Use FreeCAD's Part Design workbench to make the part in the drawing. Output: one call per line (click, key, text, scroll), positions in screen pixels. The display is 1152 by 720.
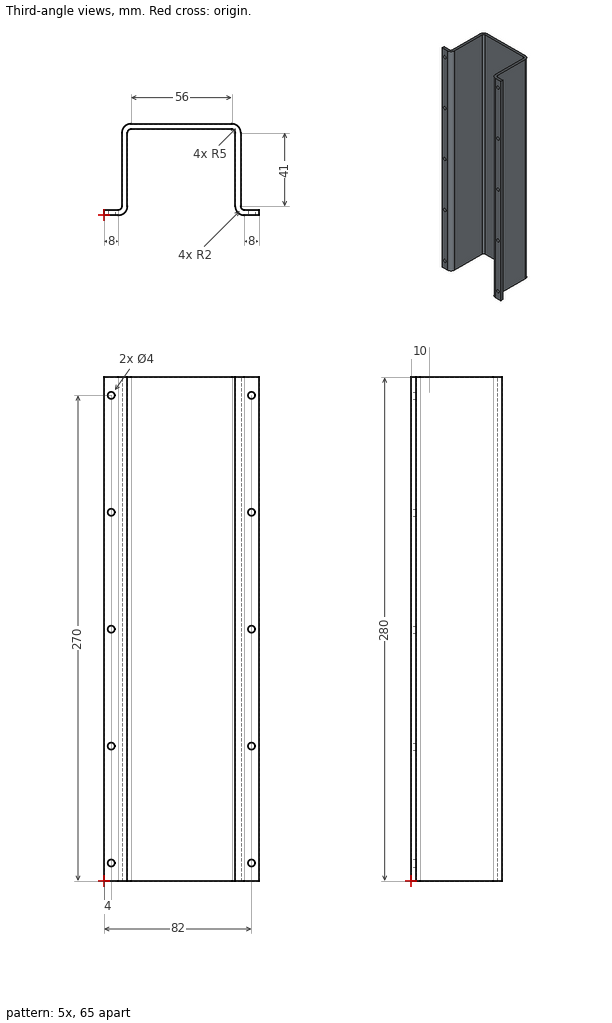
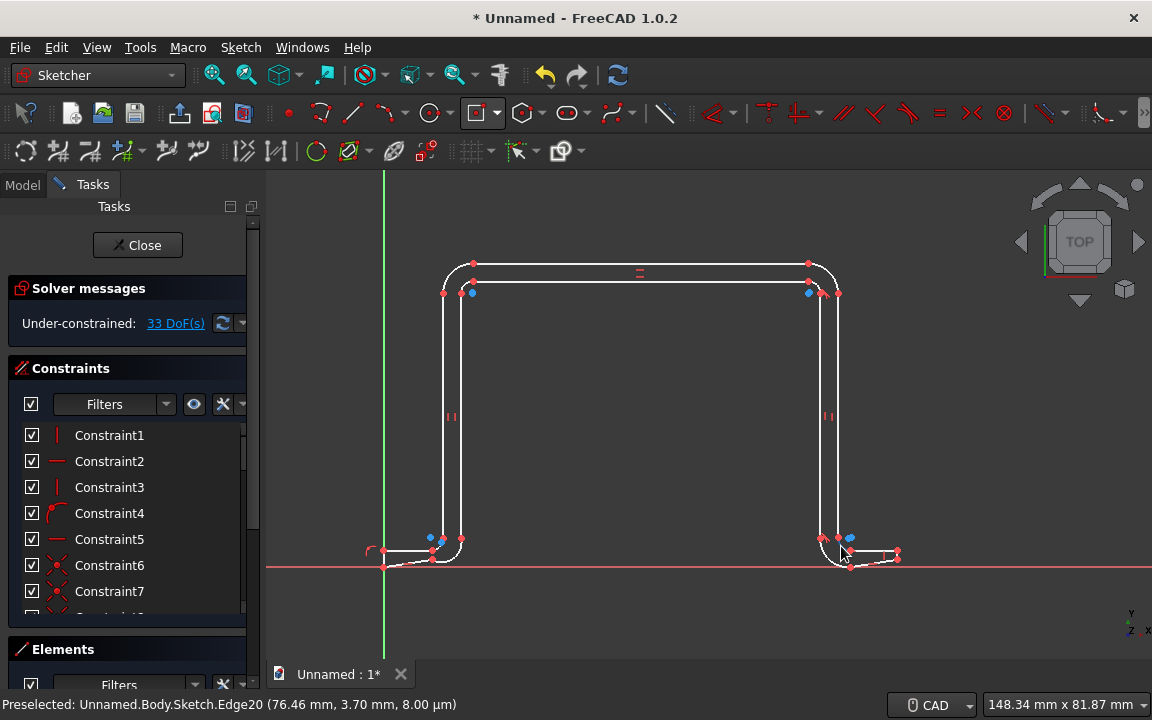
click(708, 264)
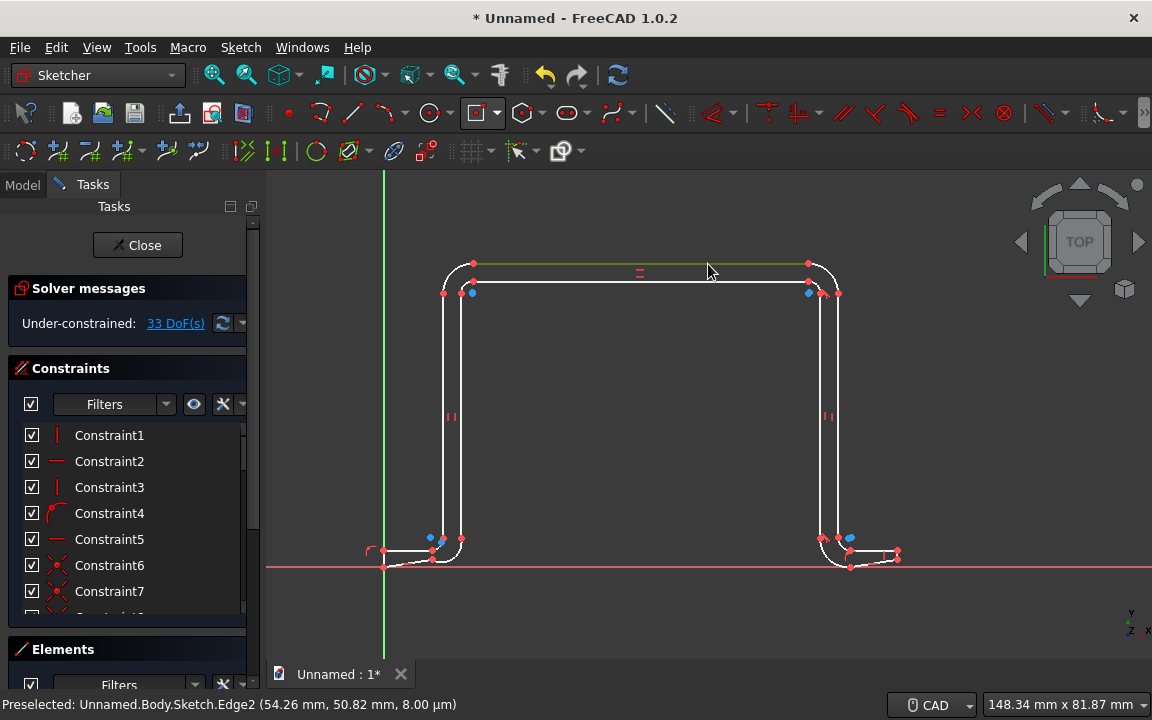
click(835, 280)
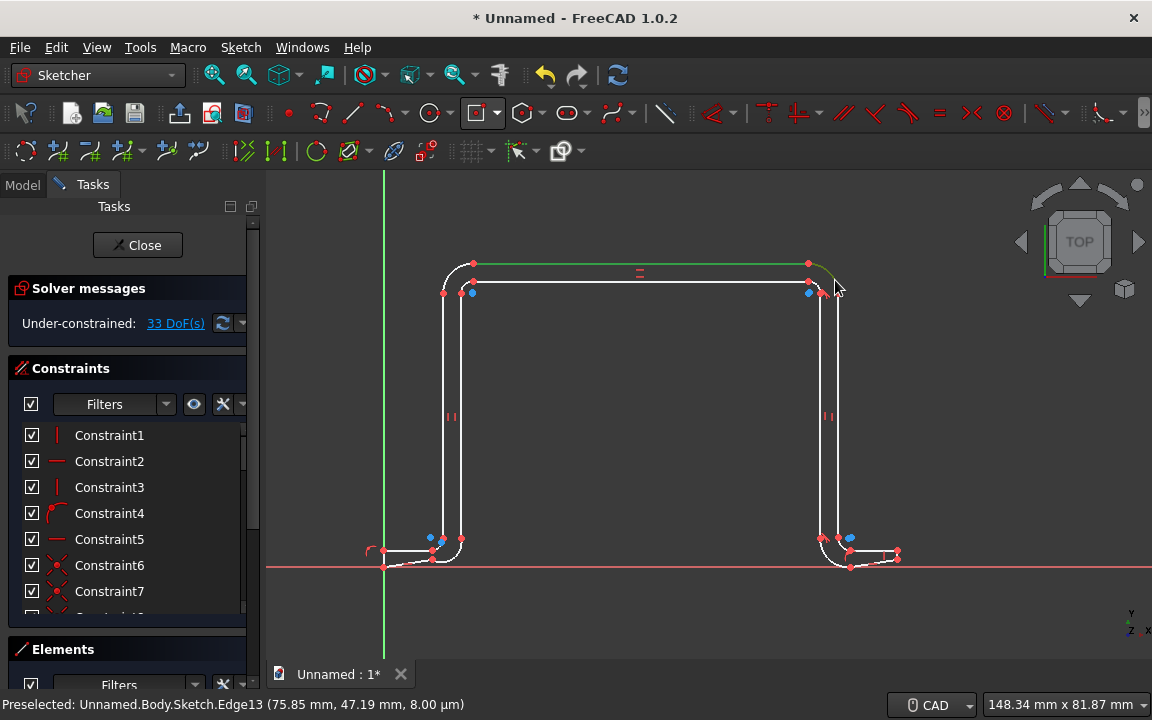
click(908, 114)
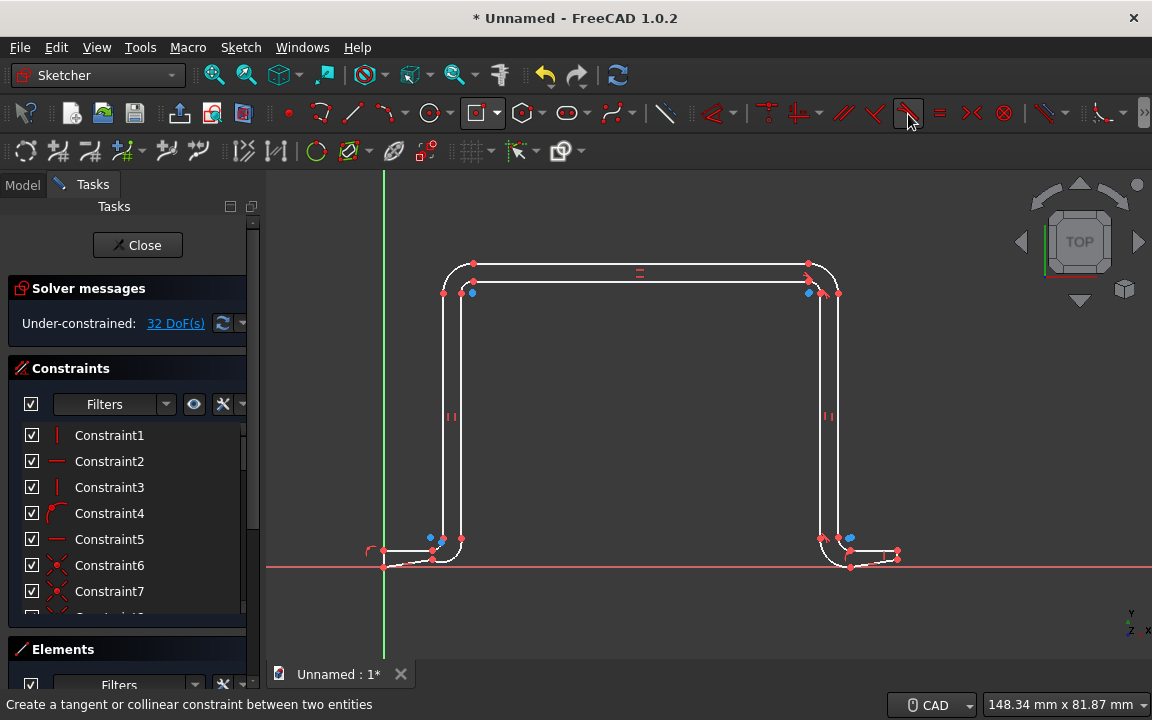
click(708, 264)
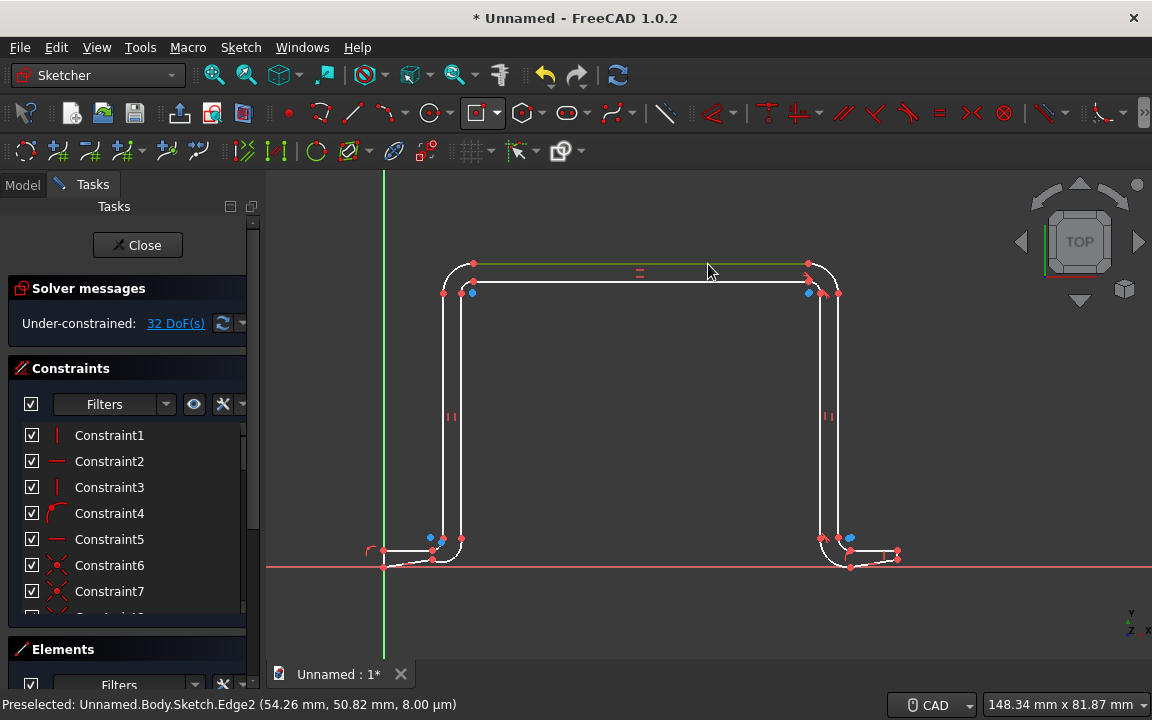
click(459, 267)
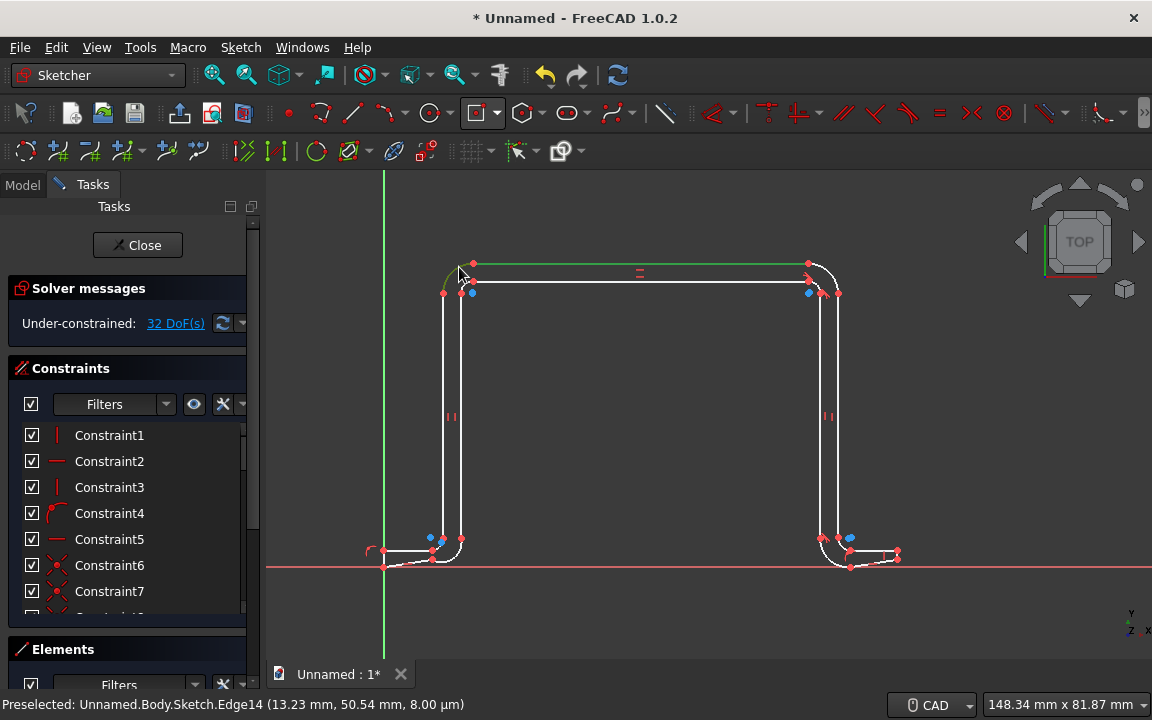
click(908, 114)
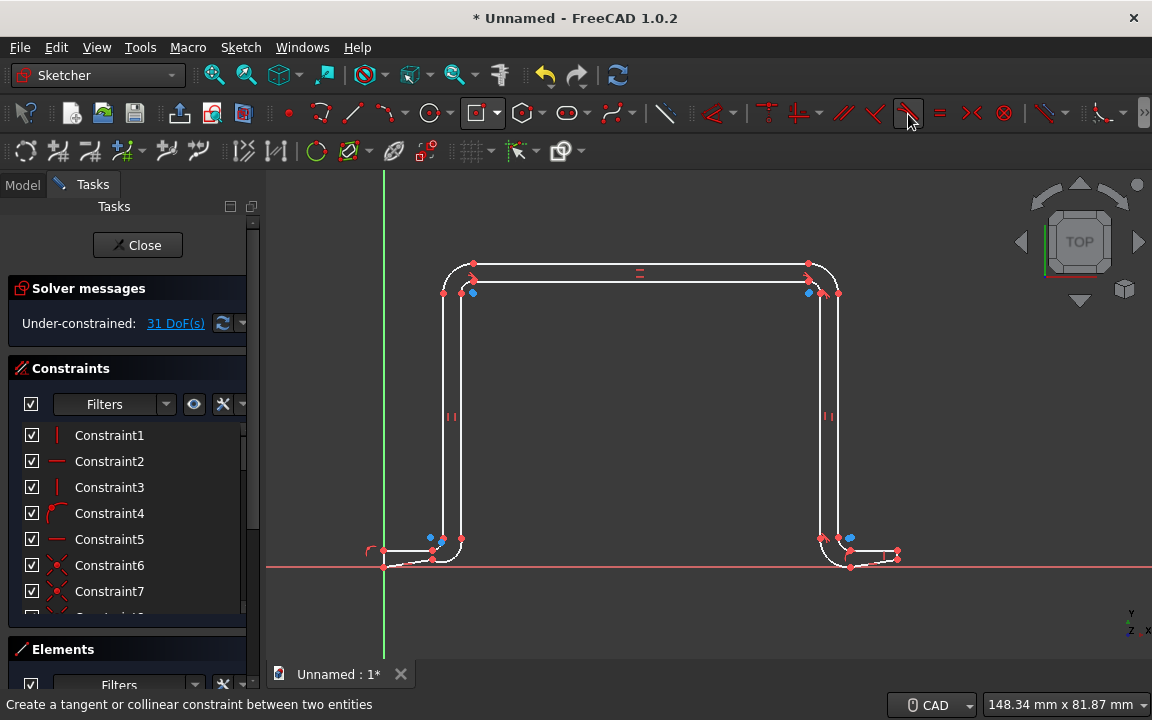
click(443, 367)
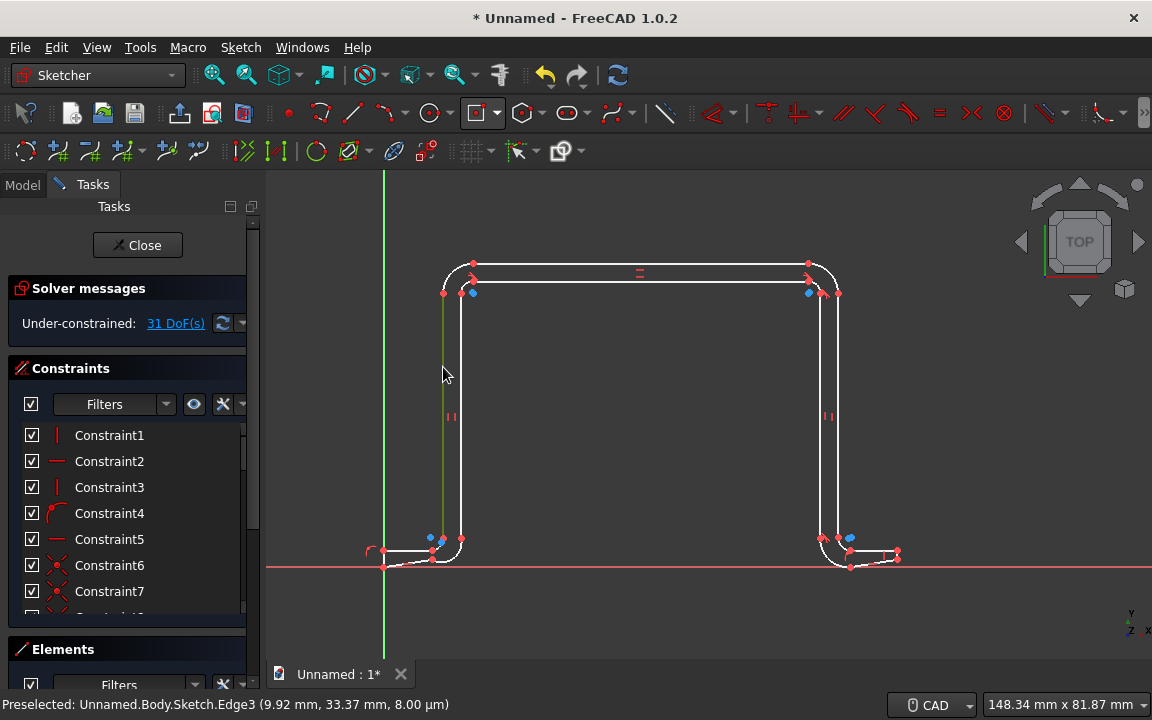
click(460, 267)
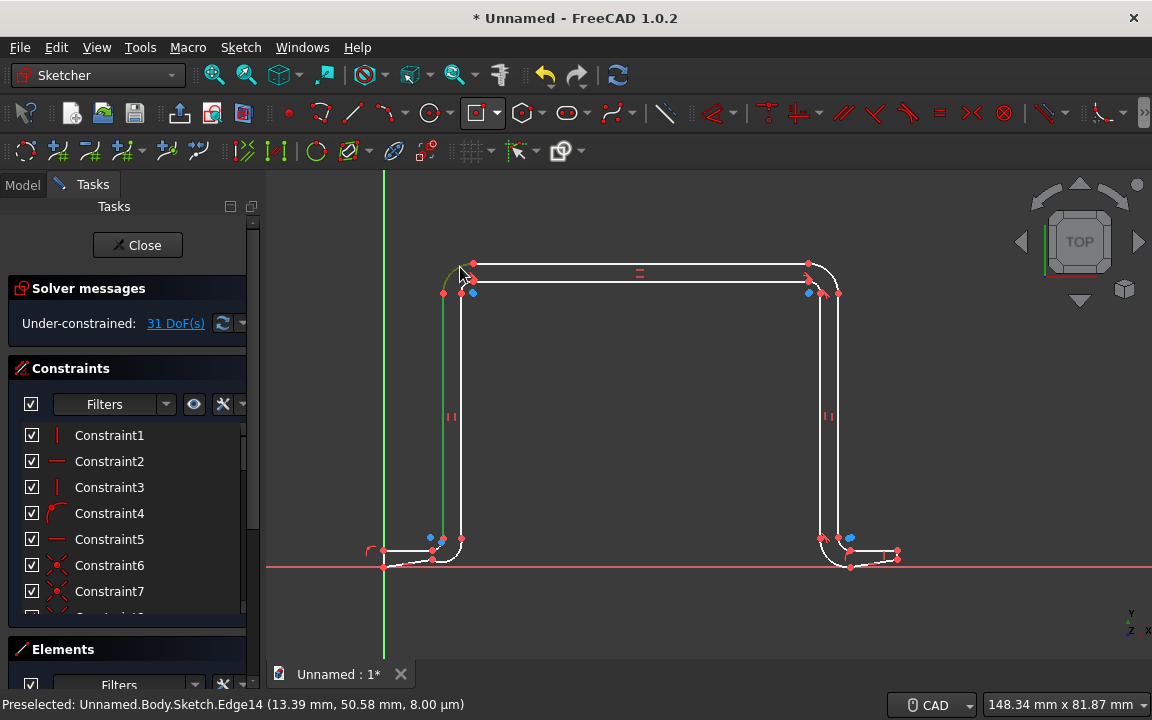
key(t)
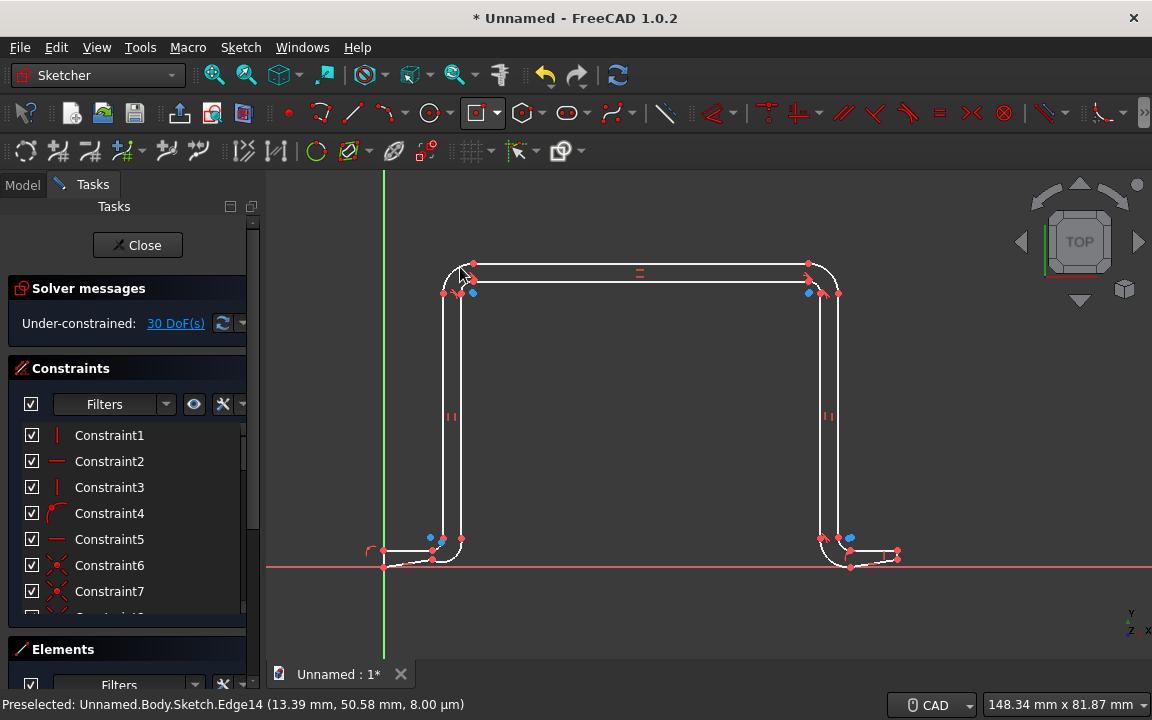
click(443, 367)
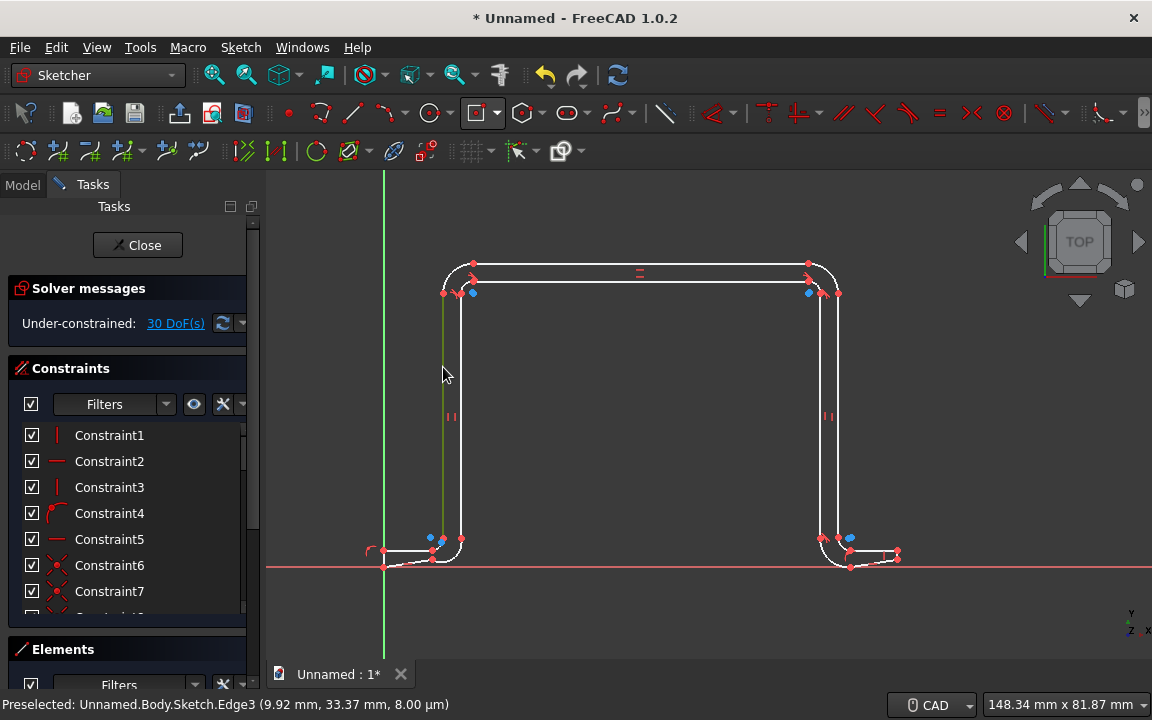
scroll(440, 547, up, 3)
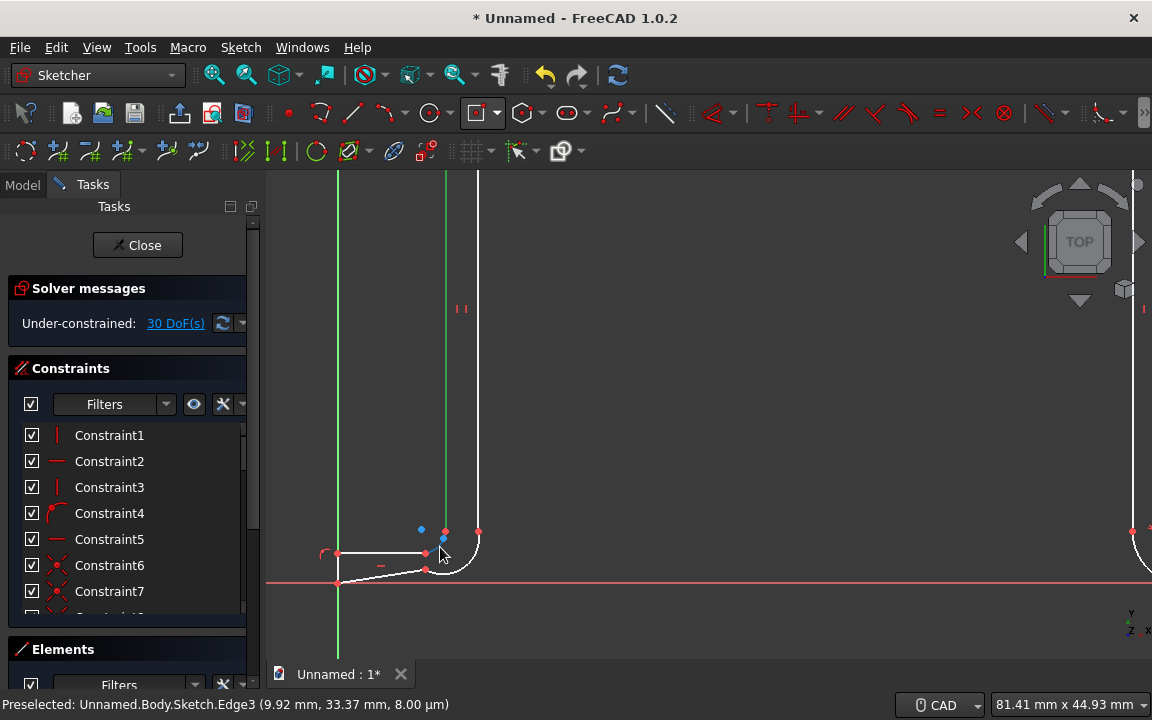
click(439, 546)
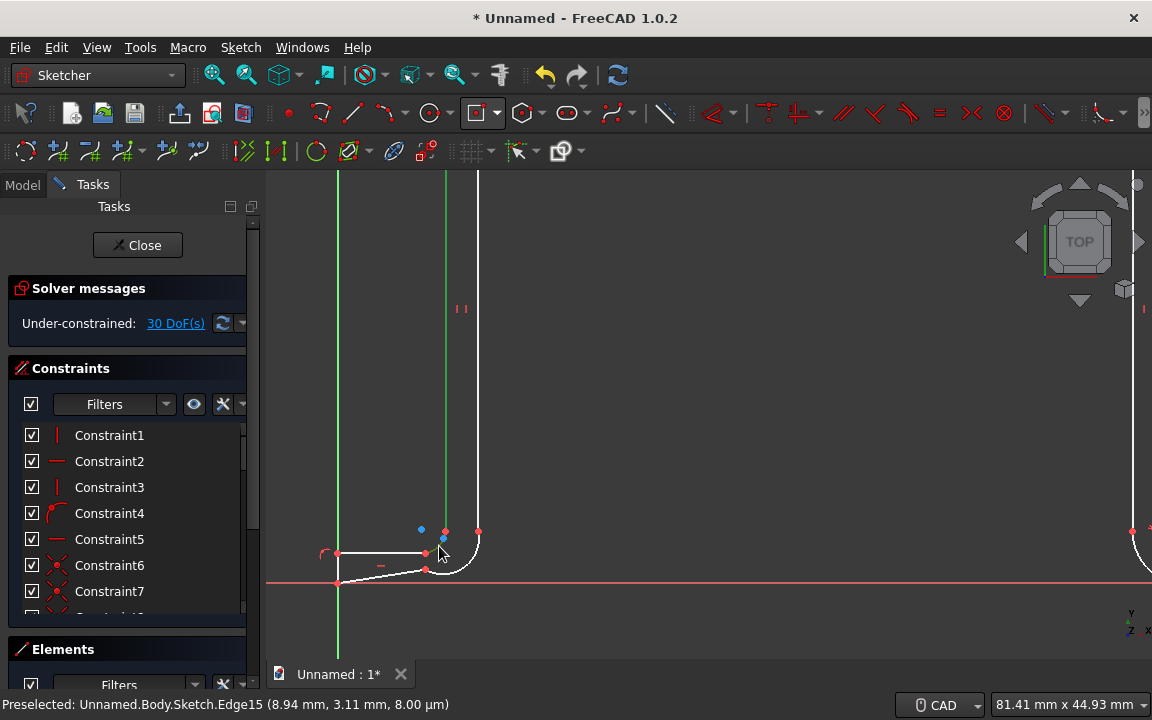
key(t)